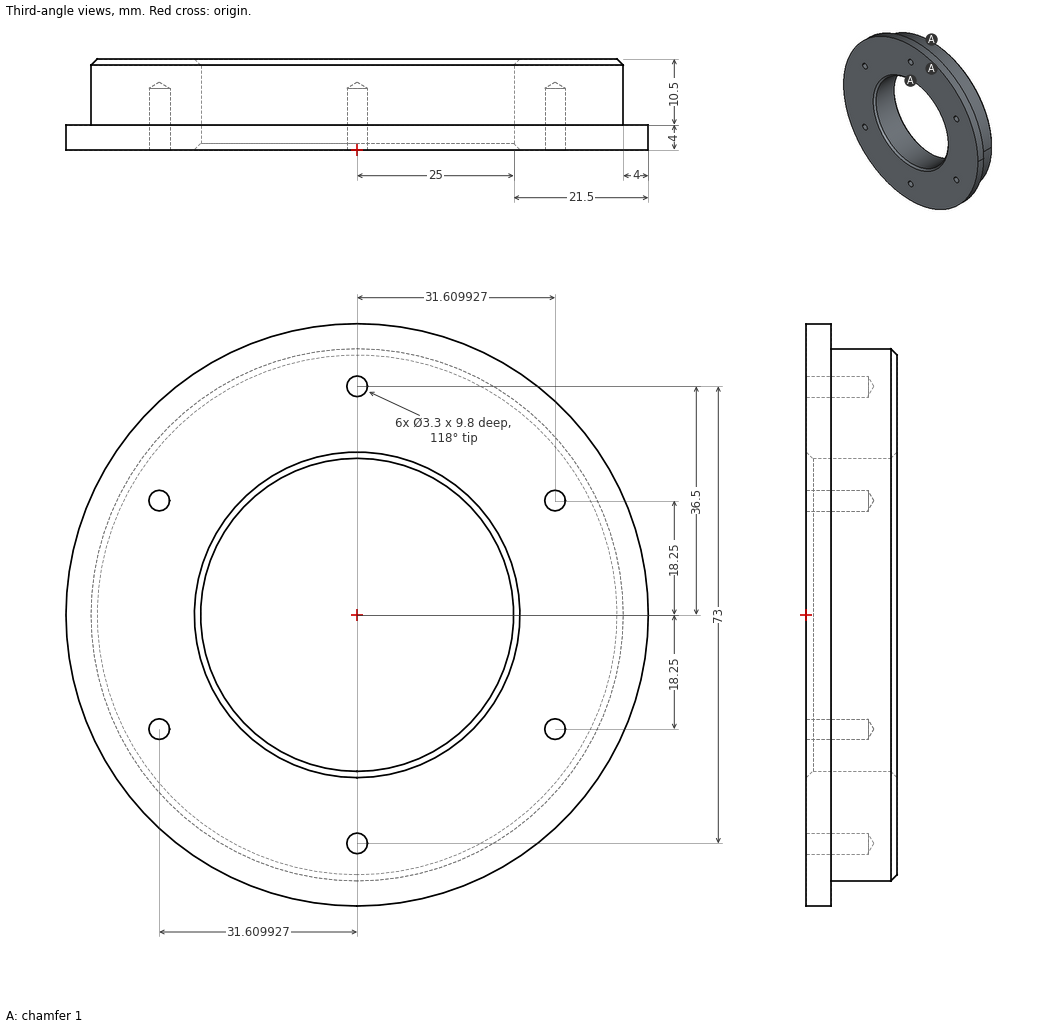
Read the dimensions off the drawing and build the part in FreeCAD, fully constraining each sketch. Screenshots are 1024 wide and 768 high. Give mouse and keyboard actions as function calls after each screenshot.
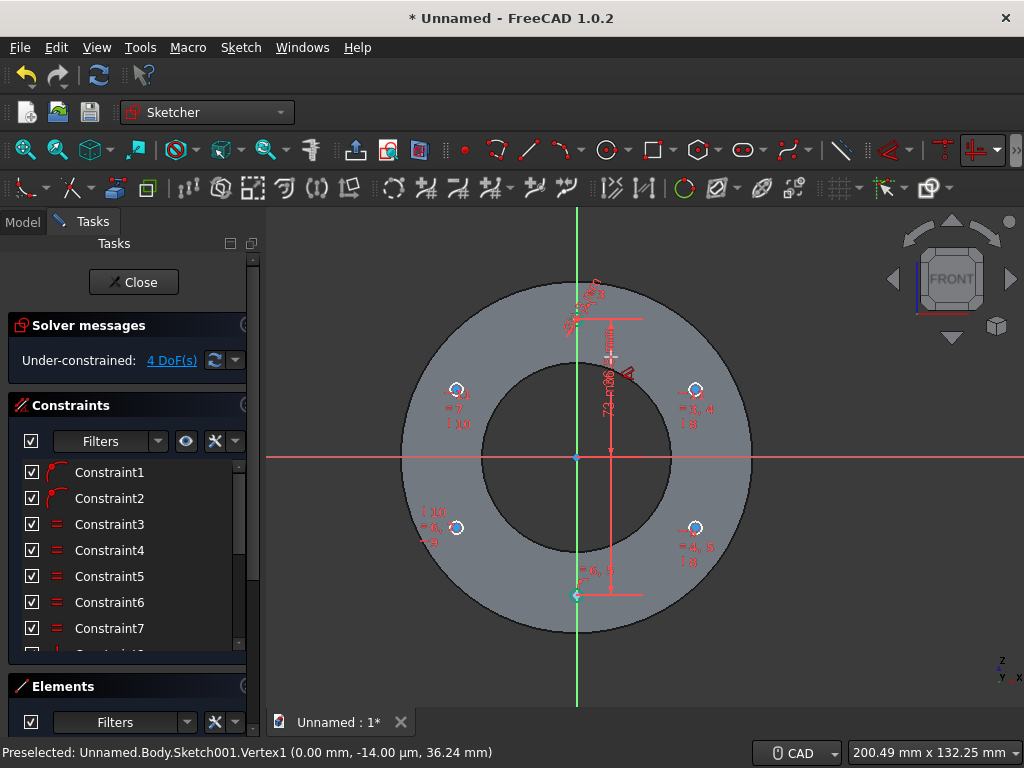
click(696, 389)
click(730, 423)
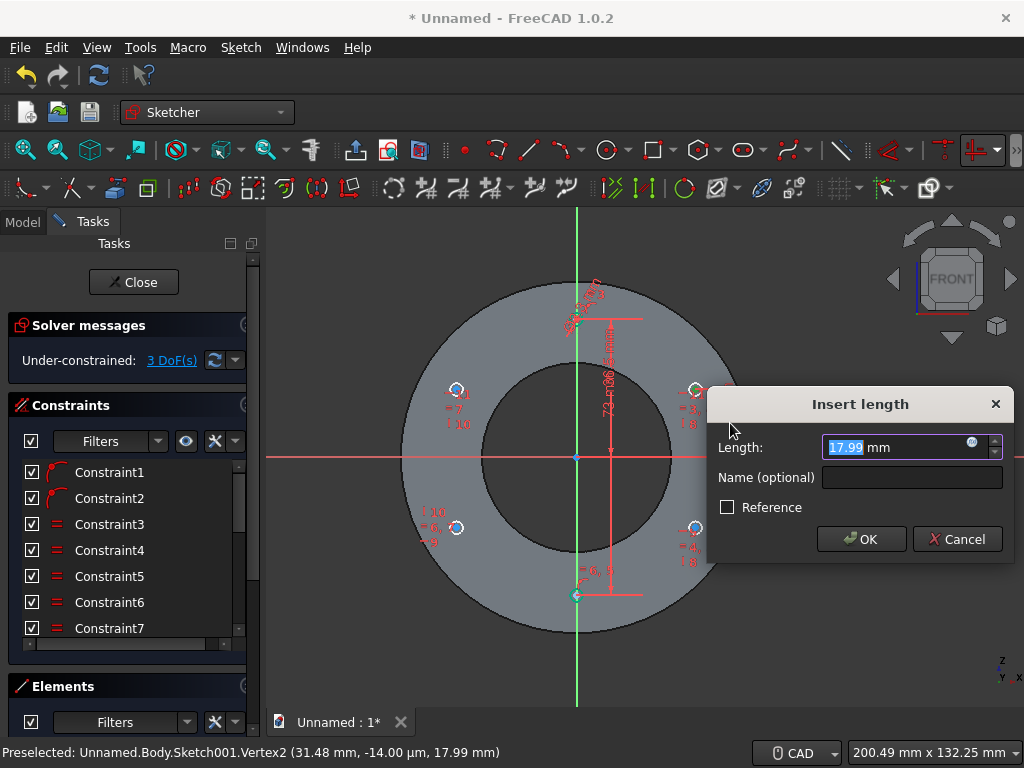
text(18.25)
key(Return)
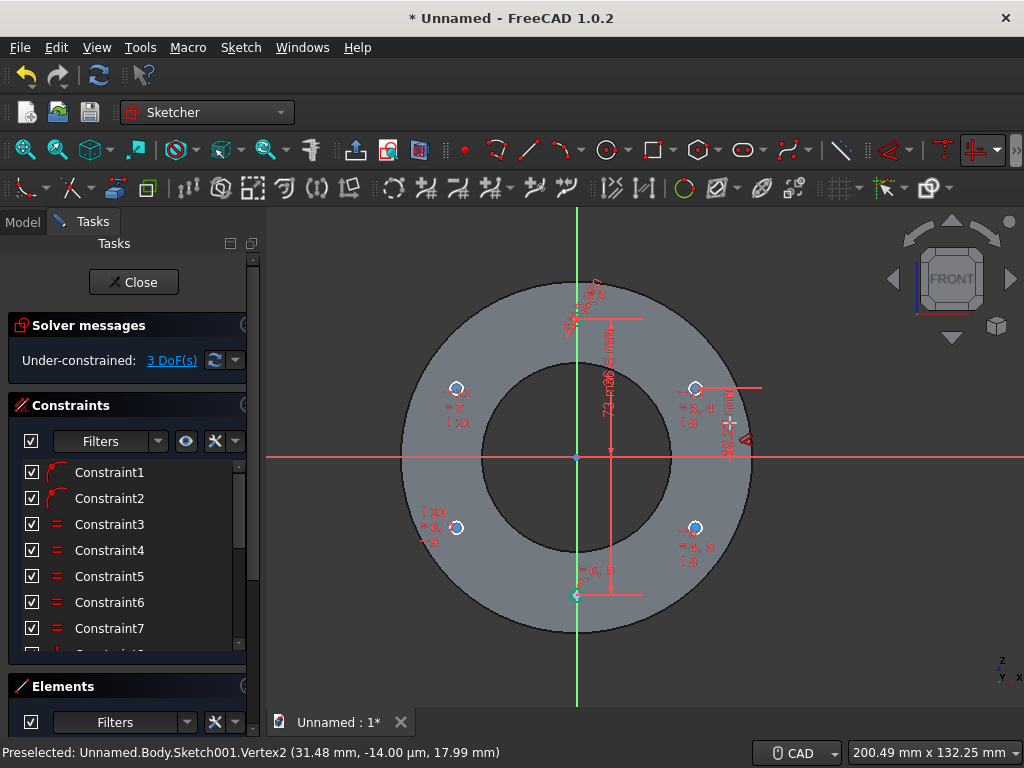
click(696, 528)
click(730, 493)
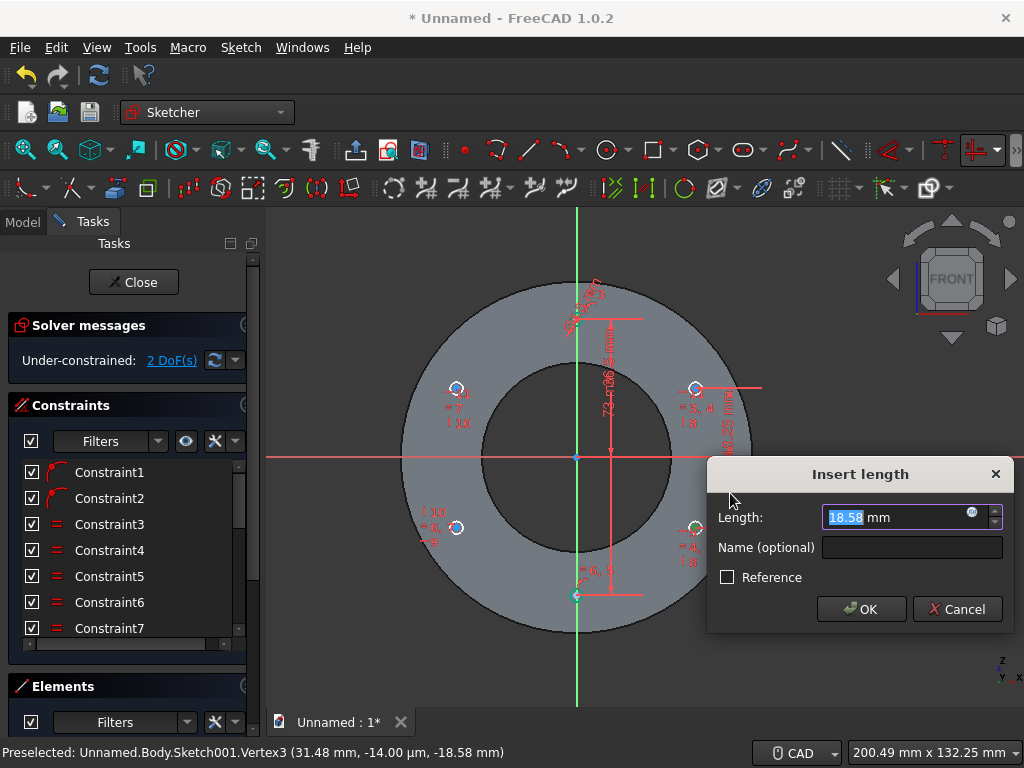
text(18.25)
key(Return)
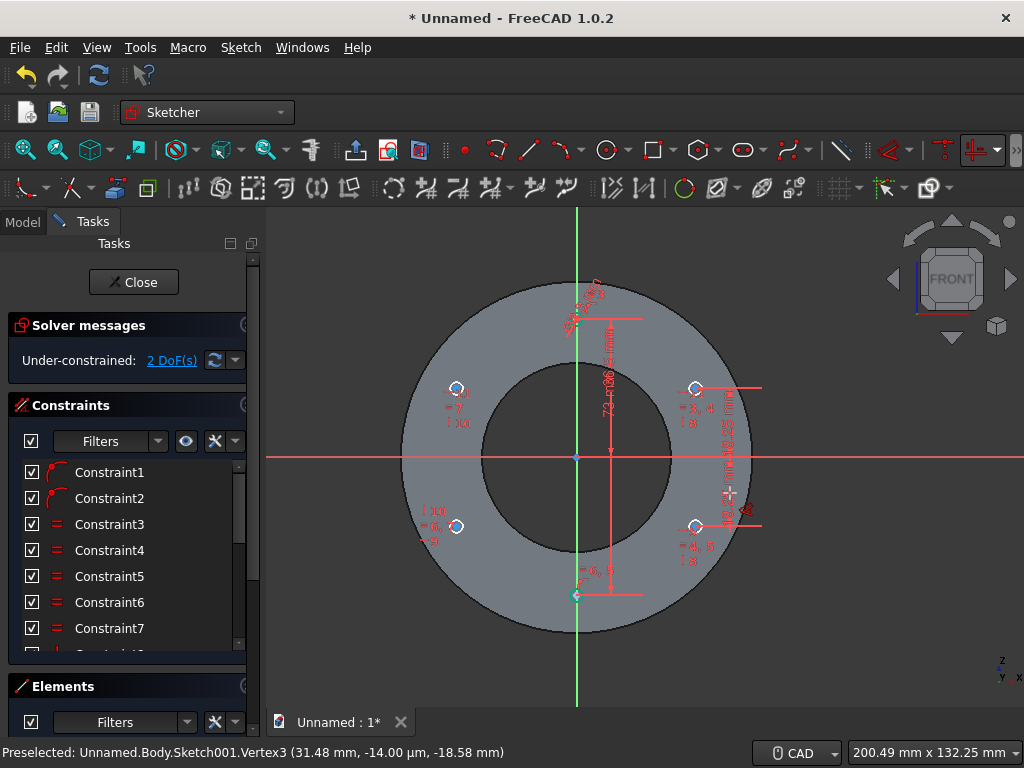
click(696, 388)
click(636, 491)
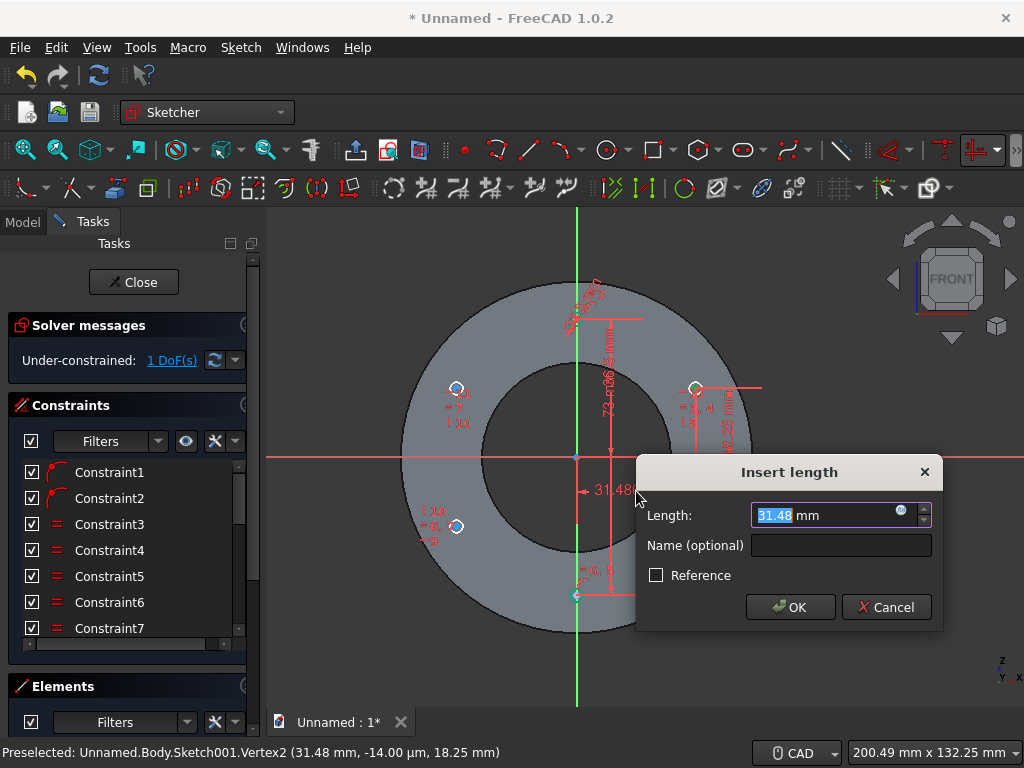
text(31.609927)
key(Return)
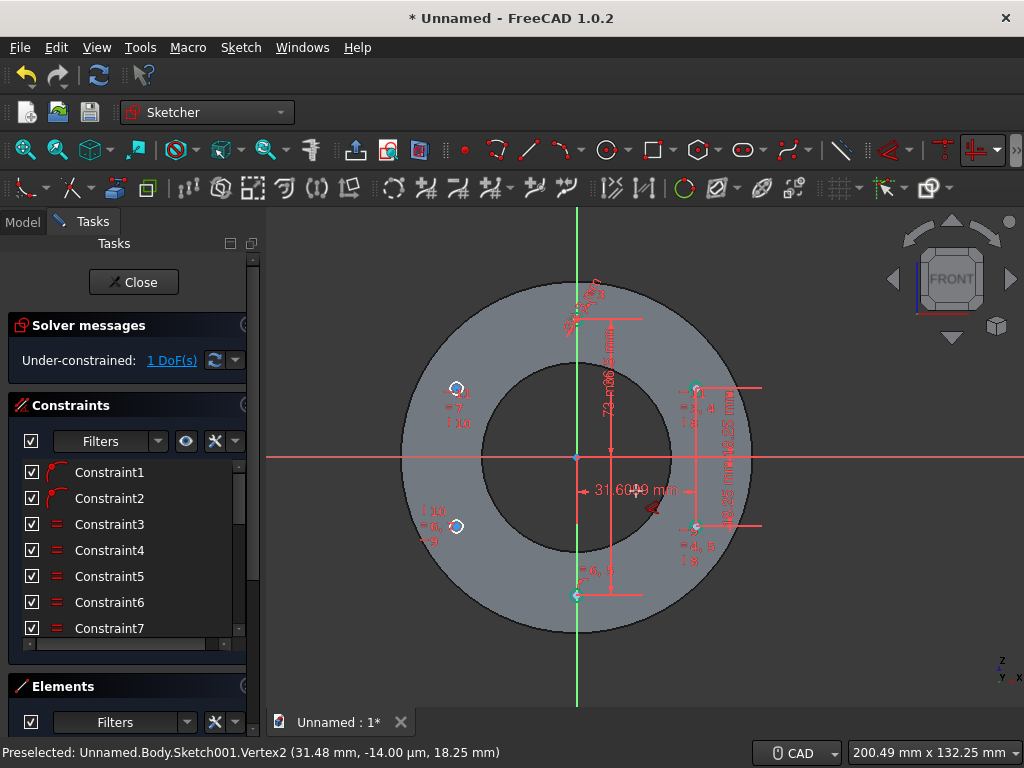
click(457, 526)
click(517, 560)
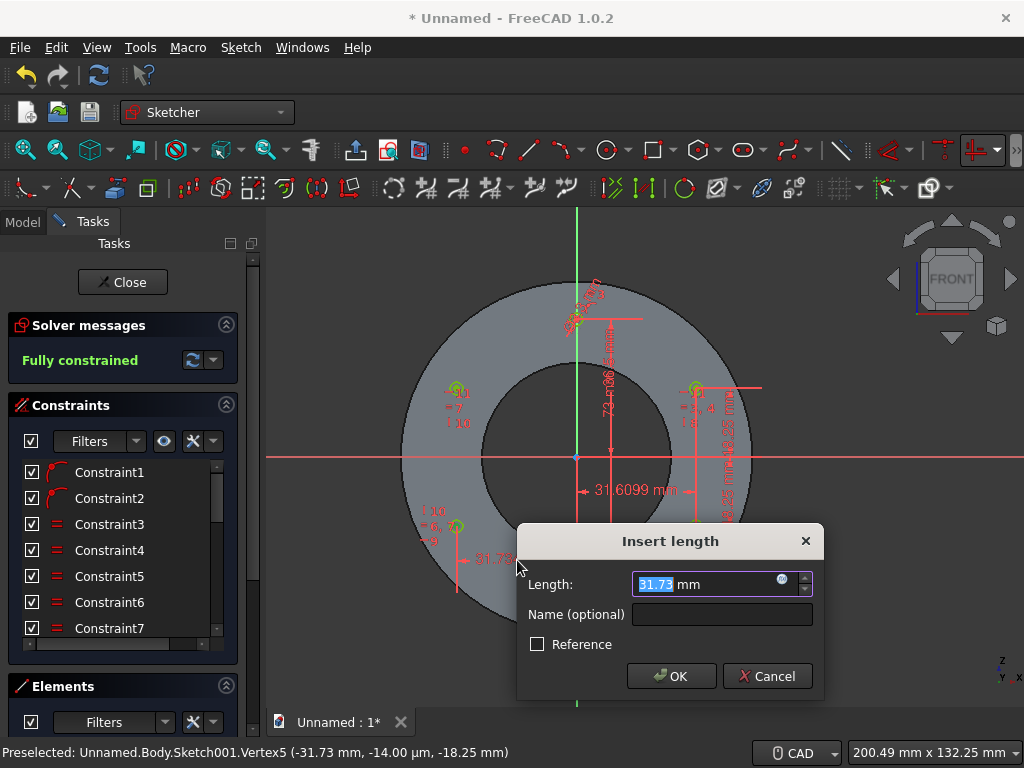
text(31.609927)
key(Return)
key(Escape)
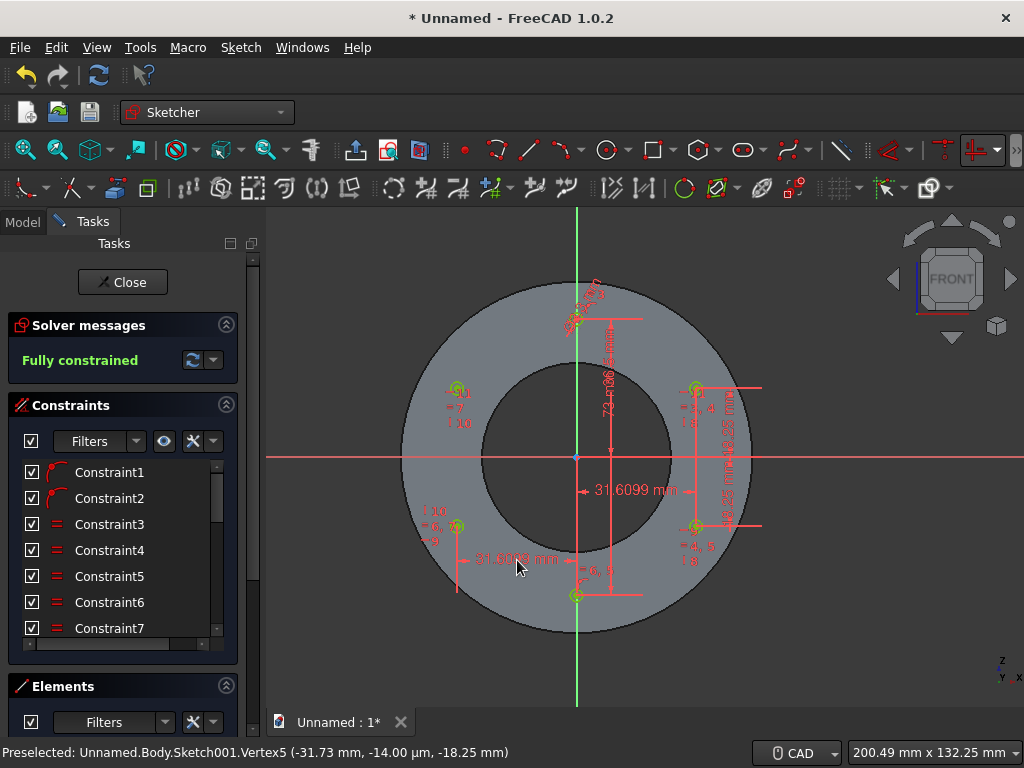
click(123, 282)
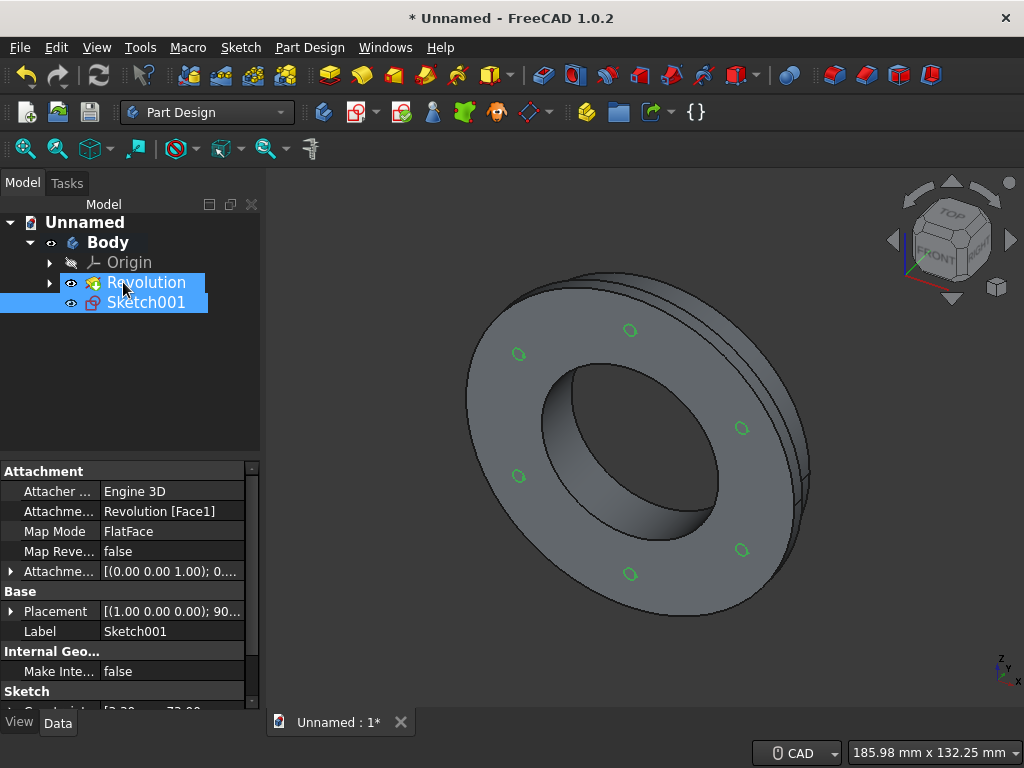
click(576, 76)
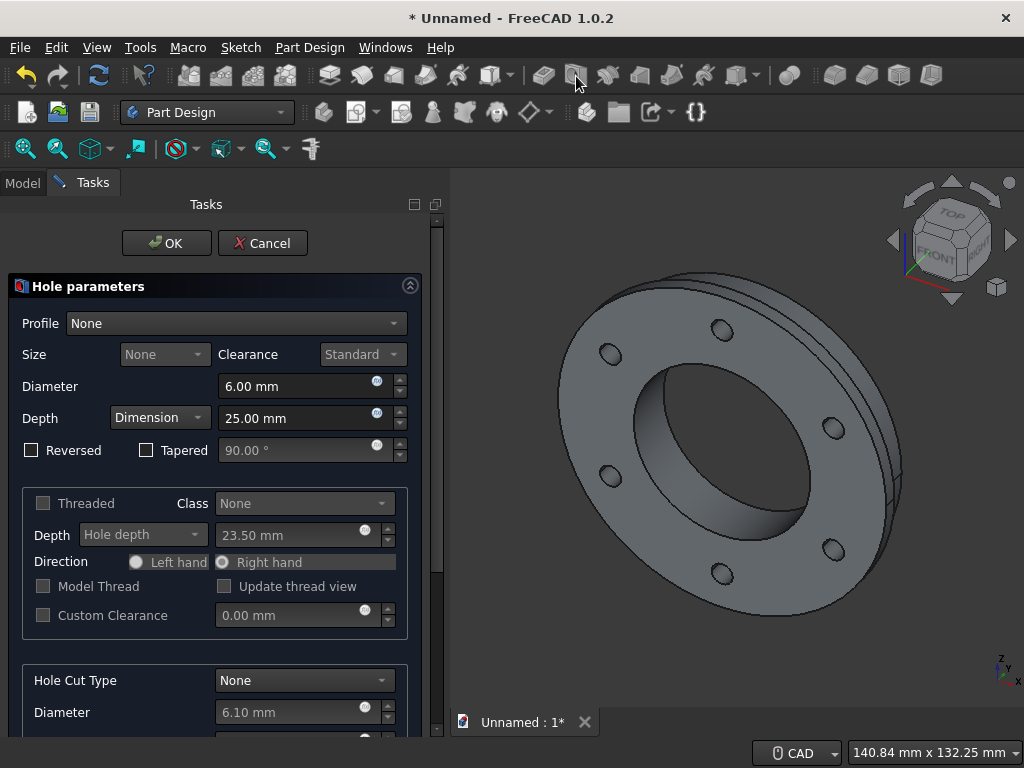
triple_click(305, 386)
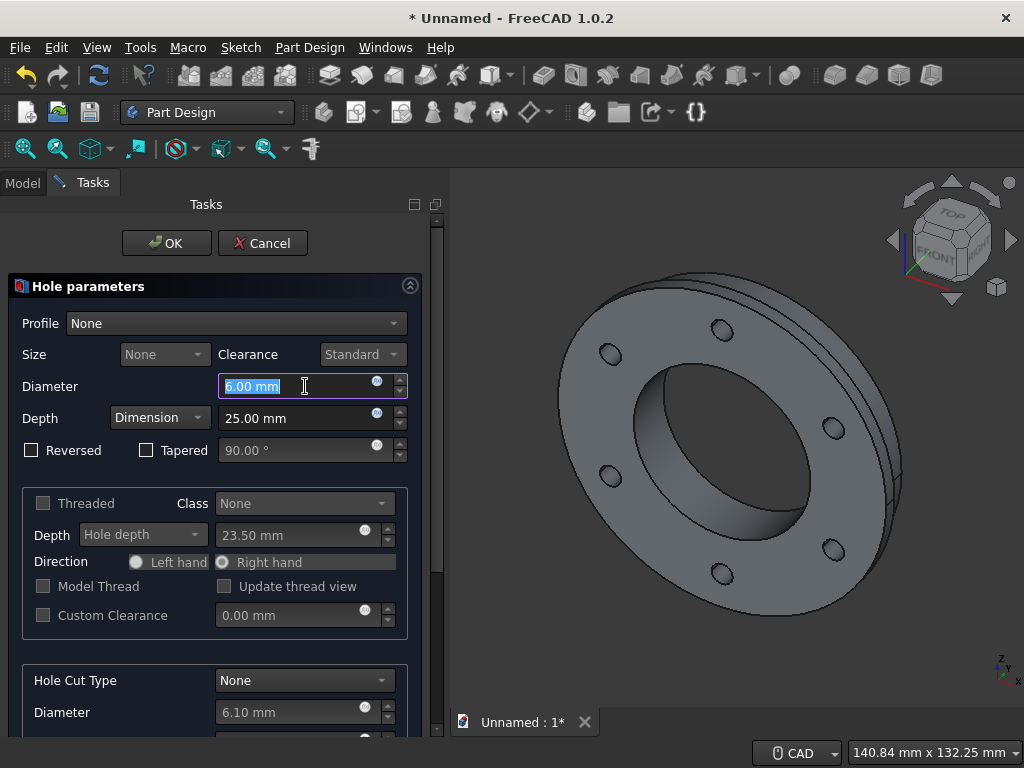
text(3.3)
key(Tab)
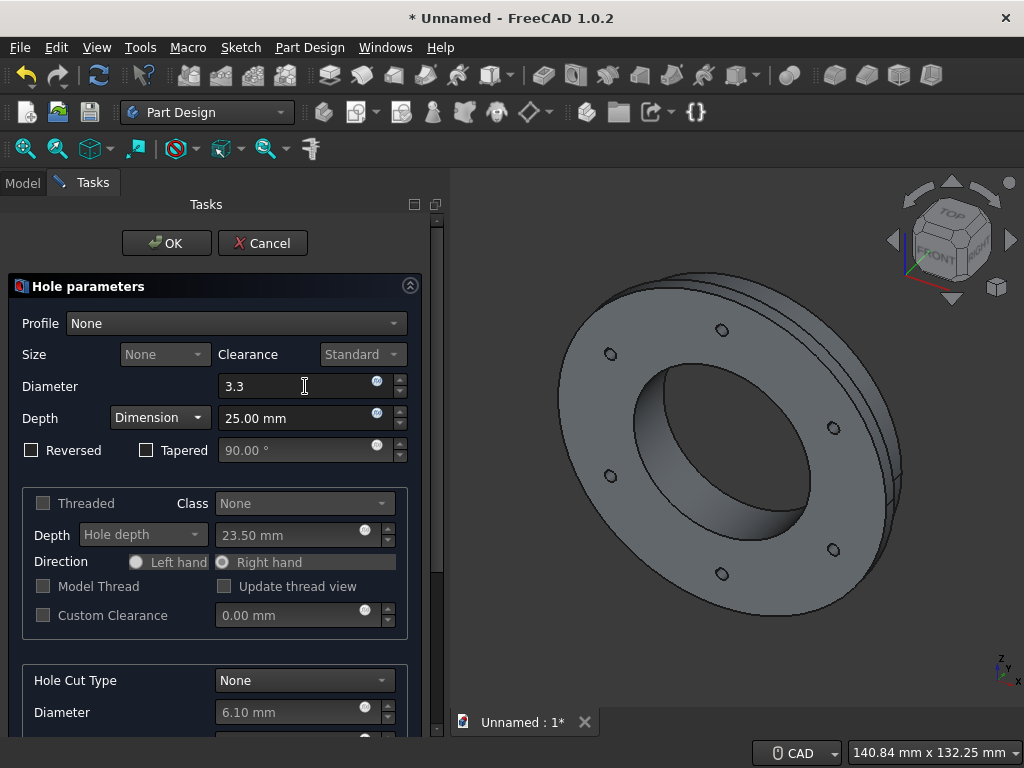
triple_click(305, 418)